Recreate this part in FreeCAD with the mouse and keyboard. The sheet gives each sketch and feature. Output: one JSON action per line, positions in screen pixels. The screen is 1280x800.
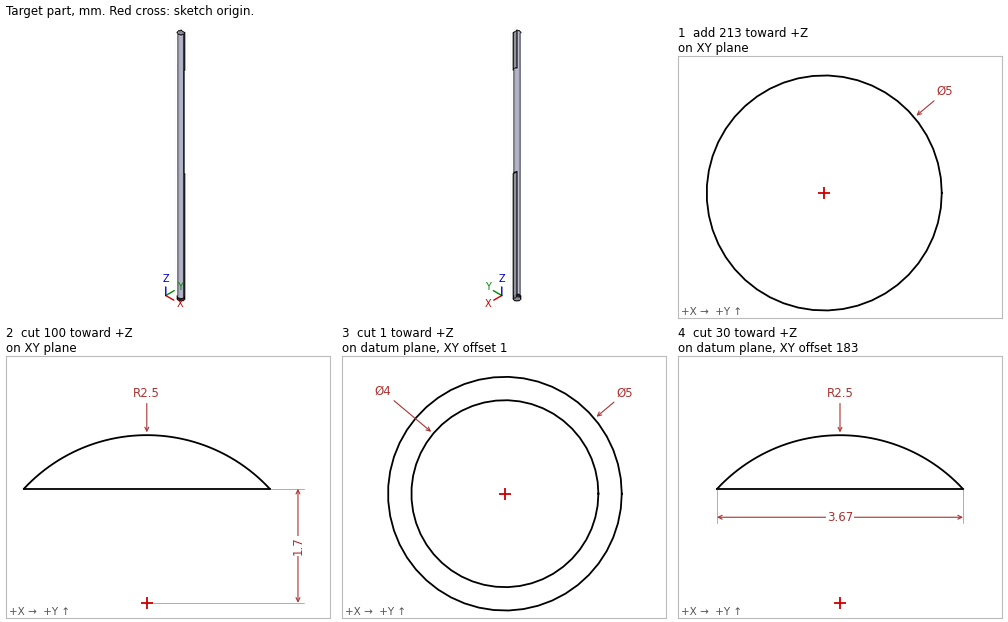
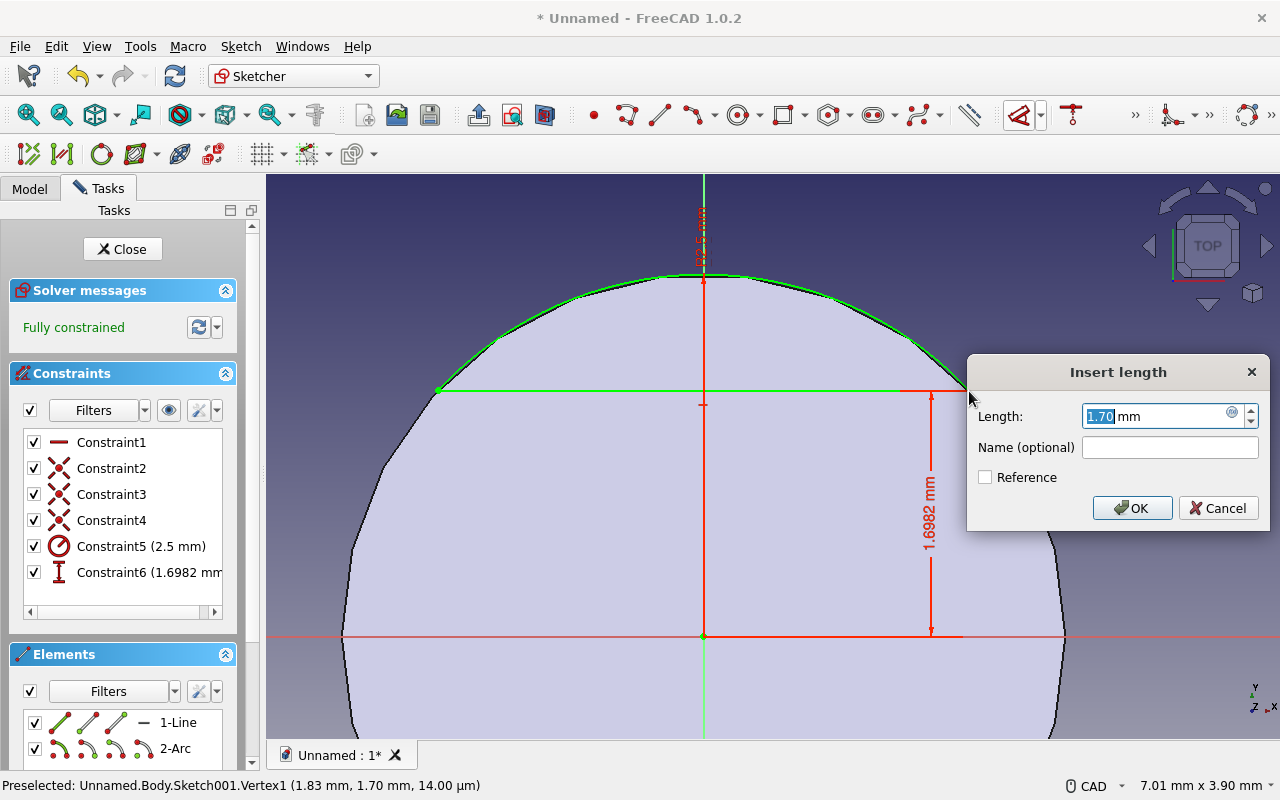
{"action": "type", "text": "1.7"}
{"action": "key", "text": "Return"}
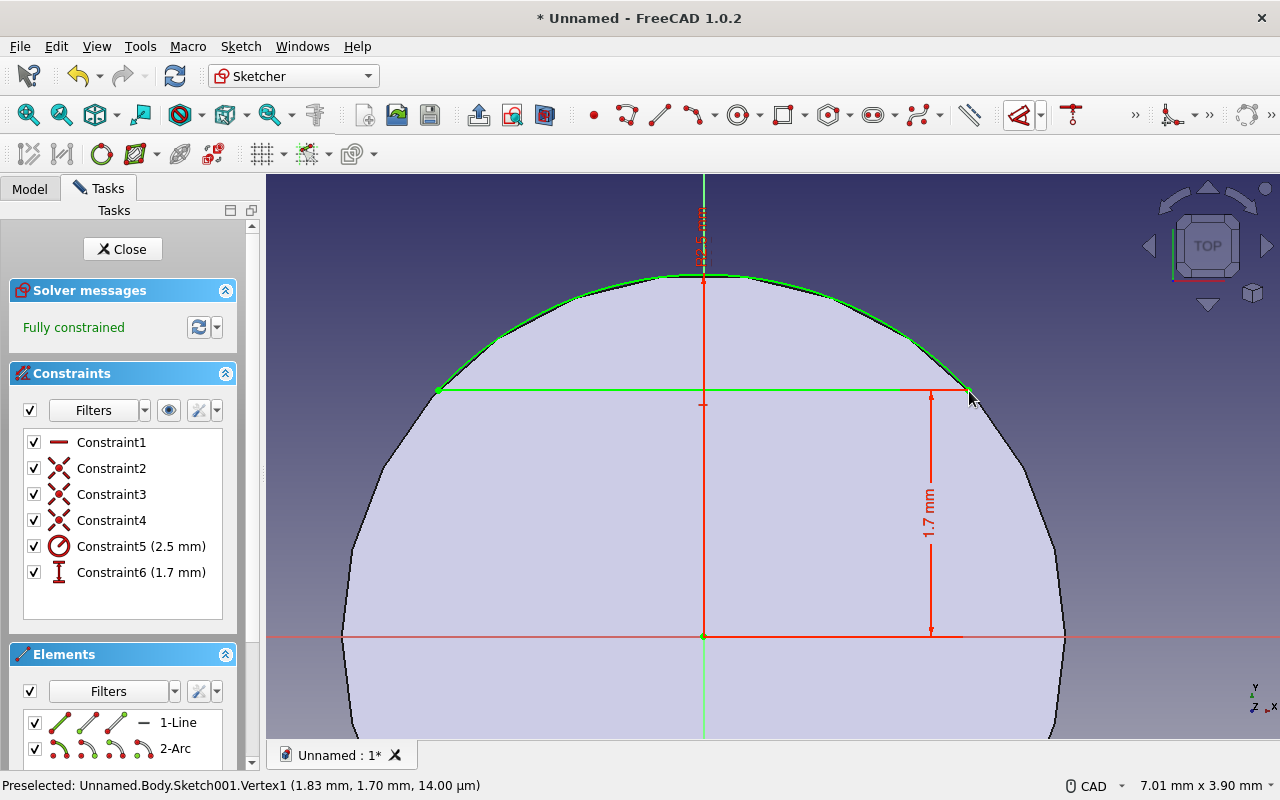
{"action": "left_click", "coordinate": [123, 249]}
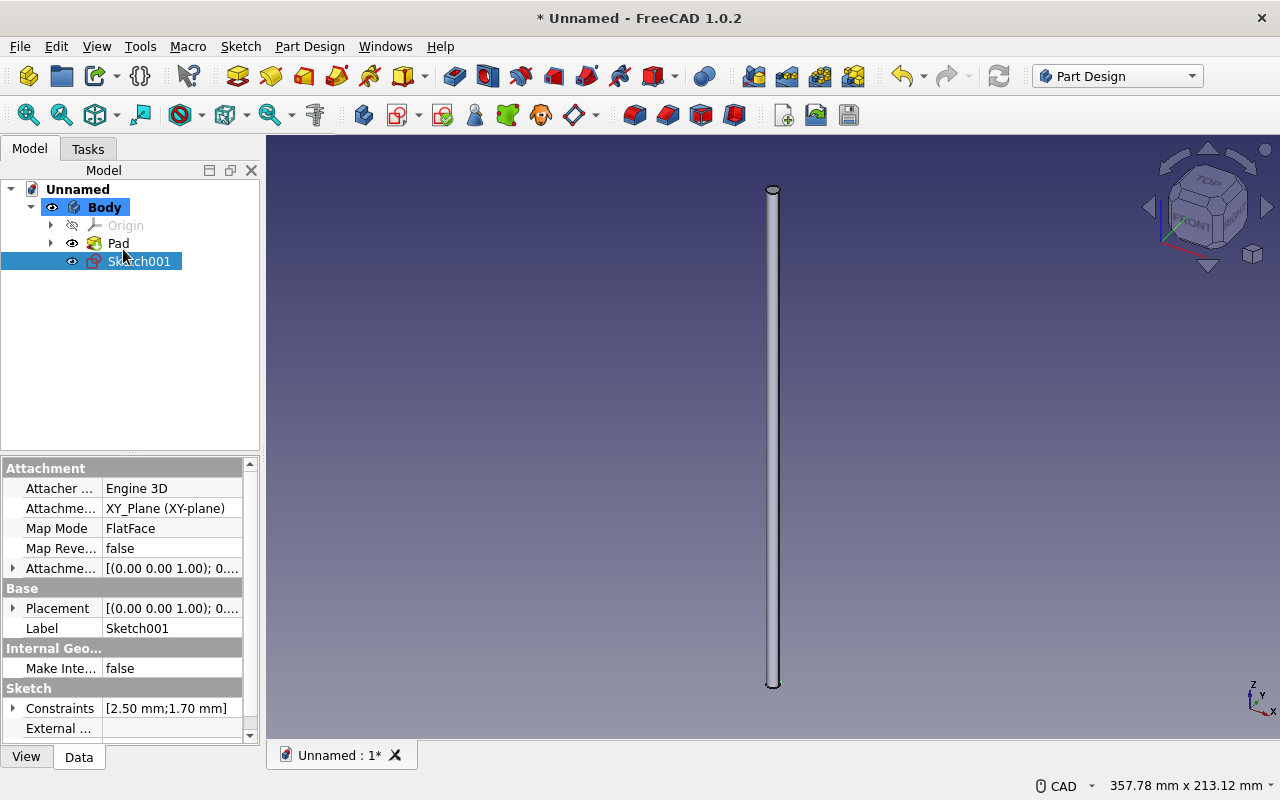
{"action": "left_click", "coordinate": [455, 76]}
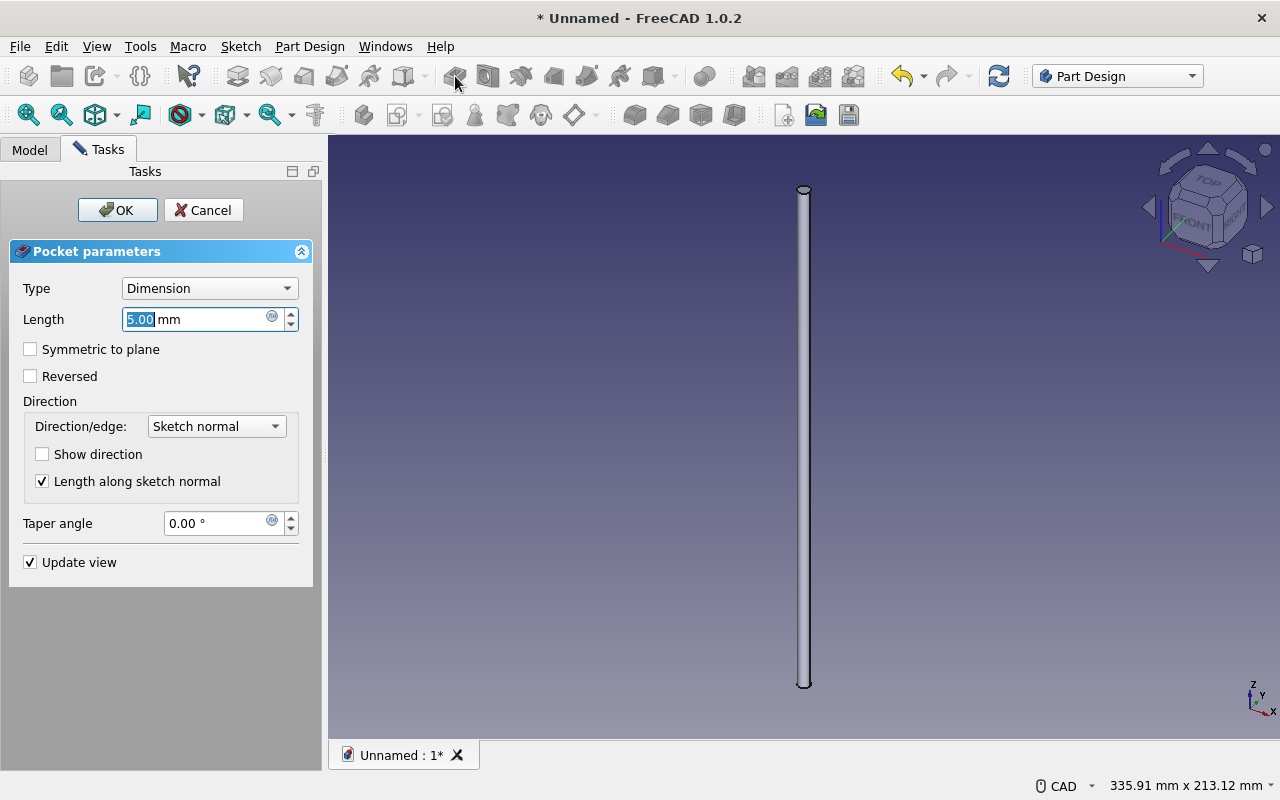
{"action": "type", "text": "100"}
{"action": "key", "text": "Tab"}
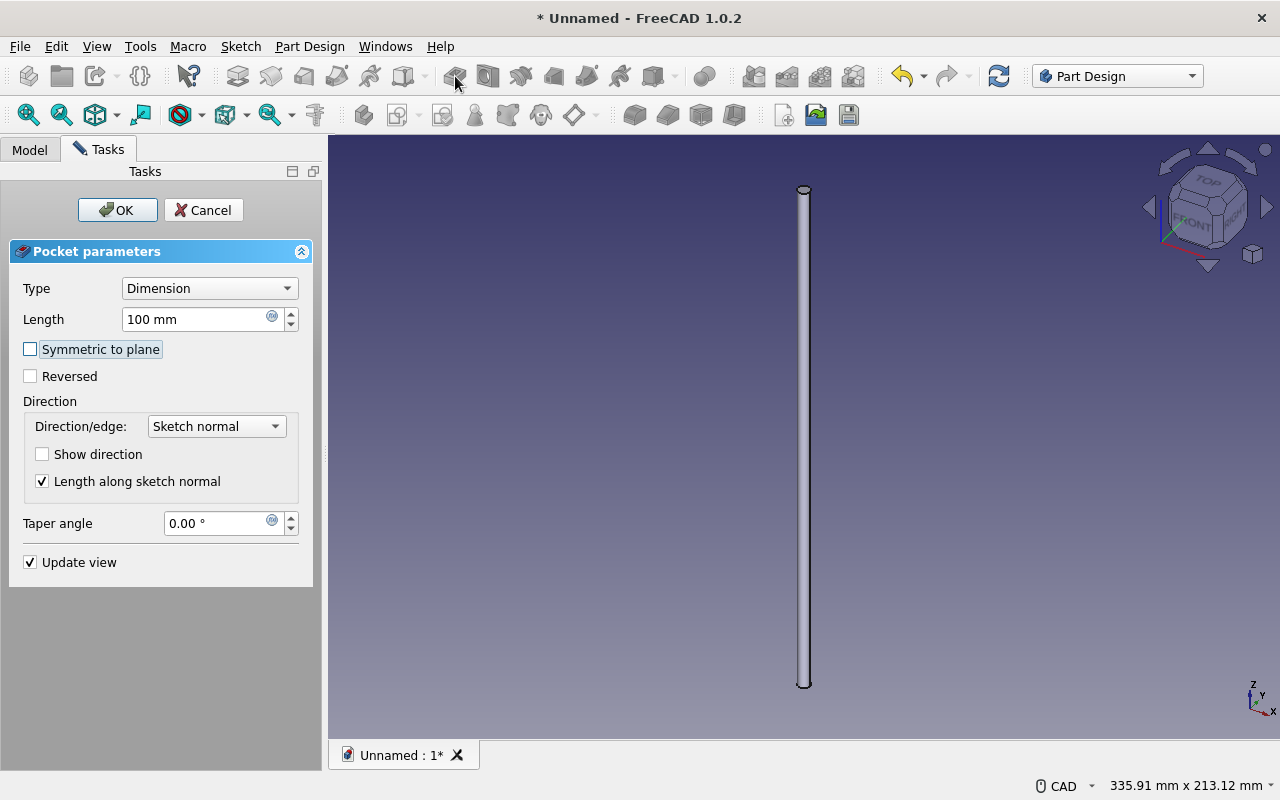
{"action": "left_click", "coordinate": [31, 376]}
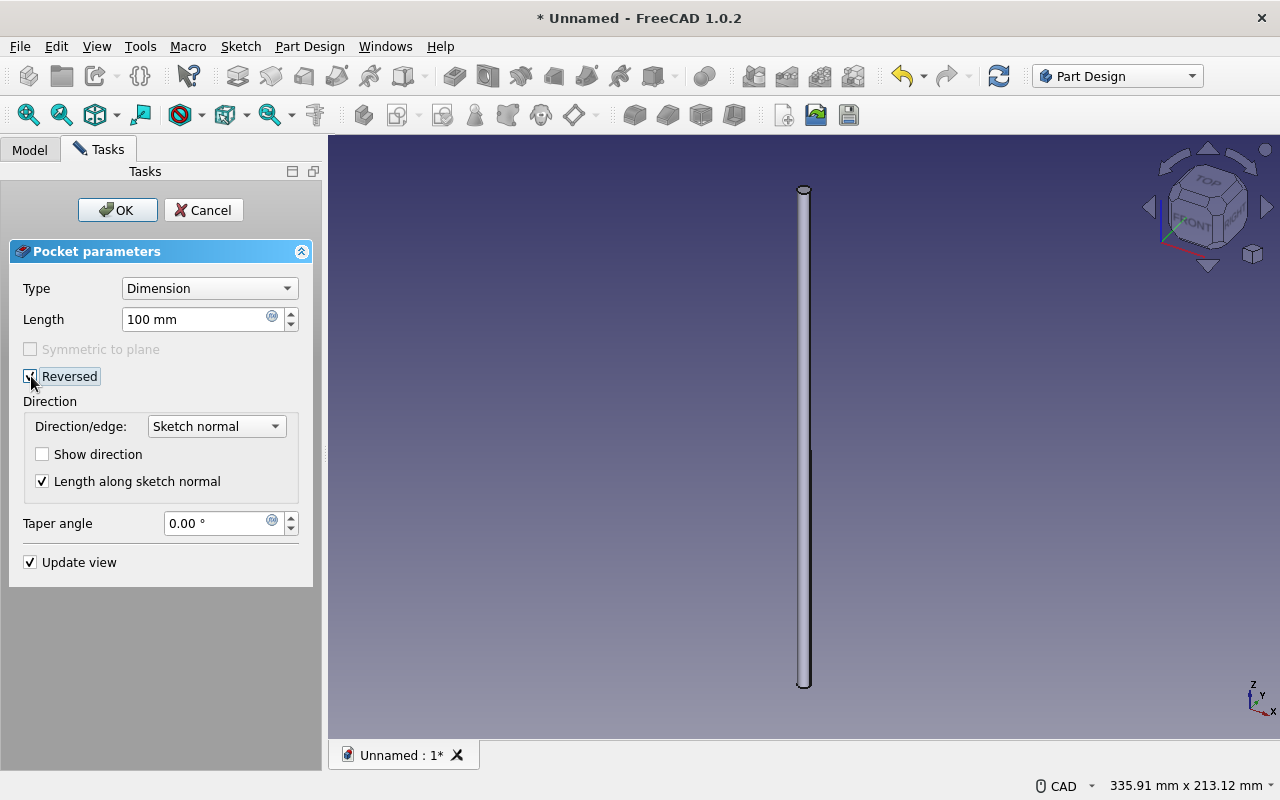
{"action": "left_click", "coordinate": [118, 210]}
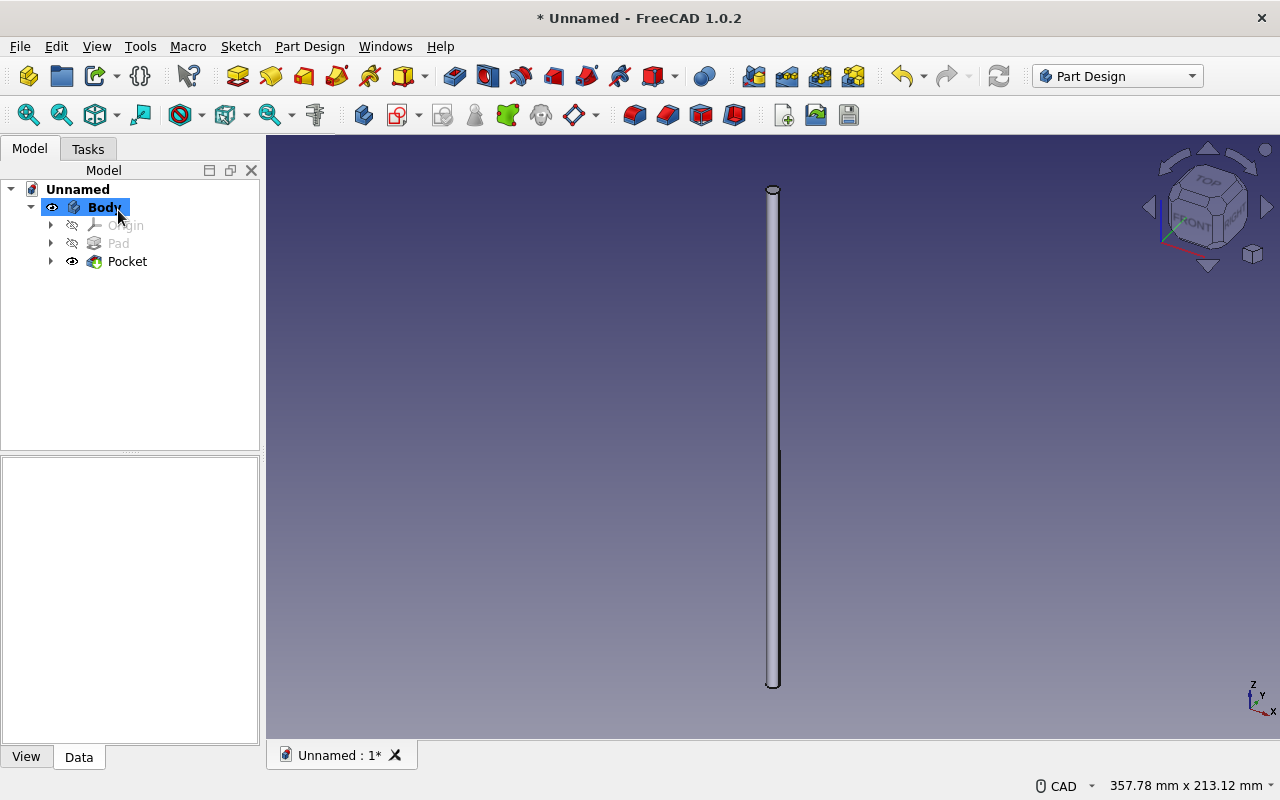
{"action": "left_click", "coordinate": [51, 225]}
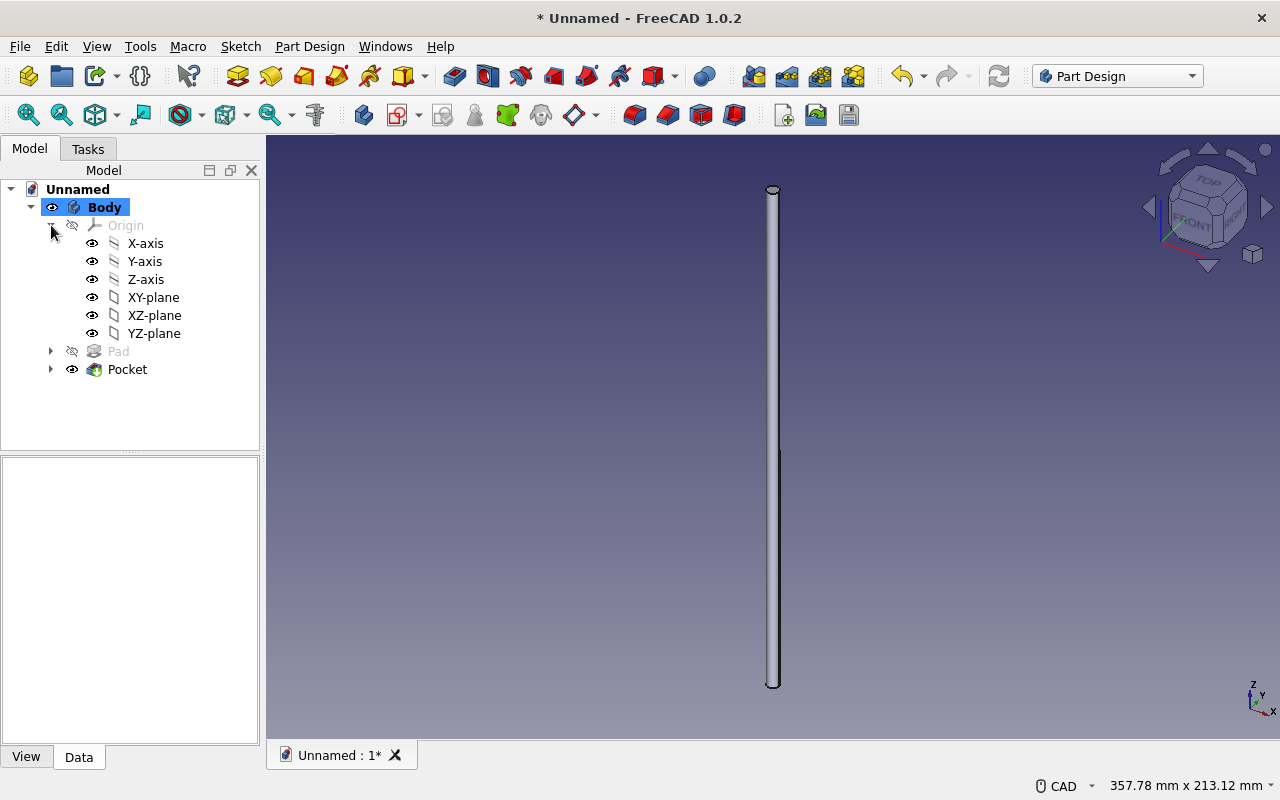
{"action": "left_click", "coordinate": [137, 297]}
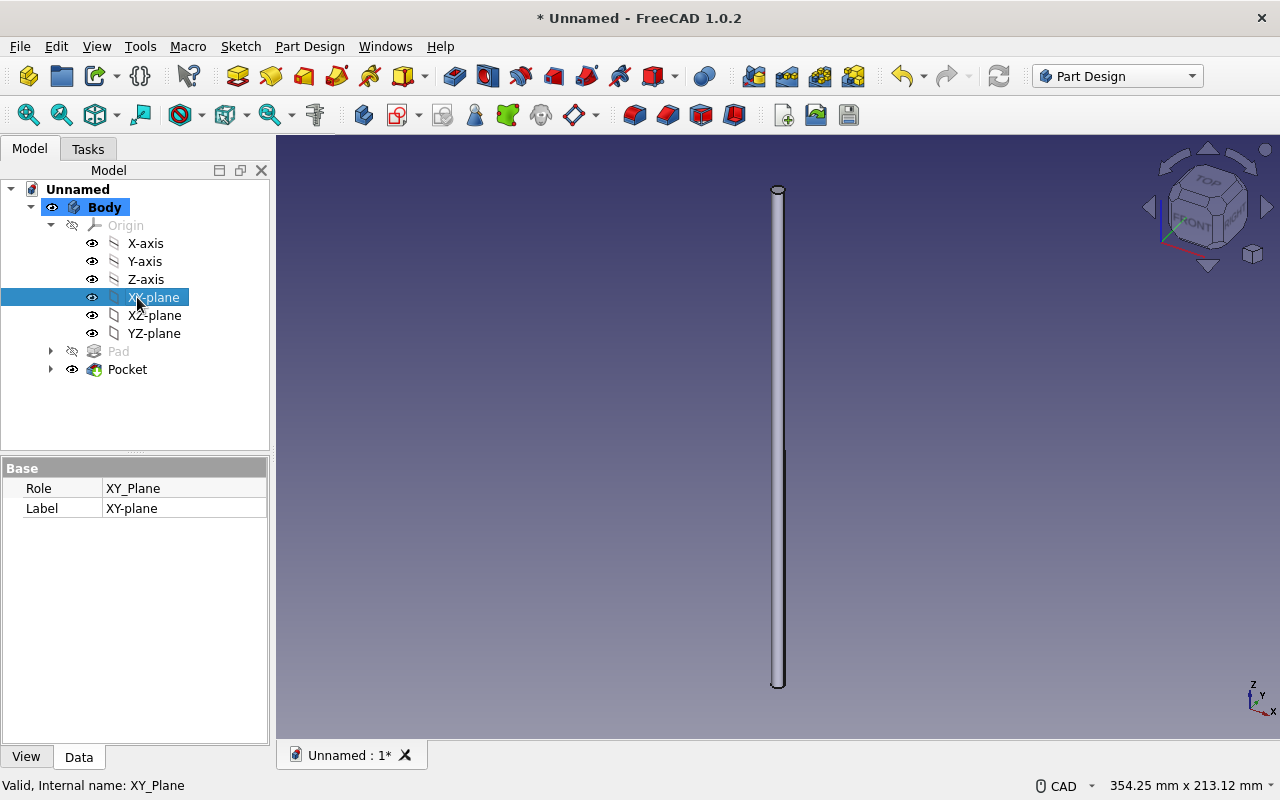
{"action": "left_click", "coordinate": [574, 116]}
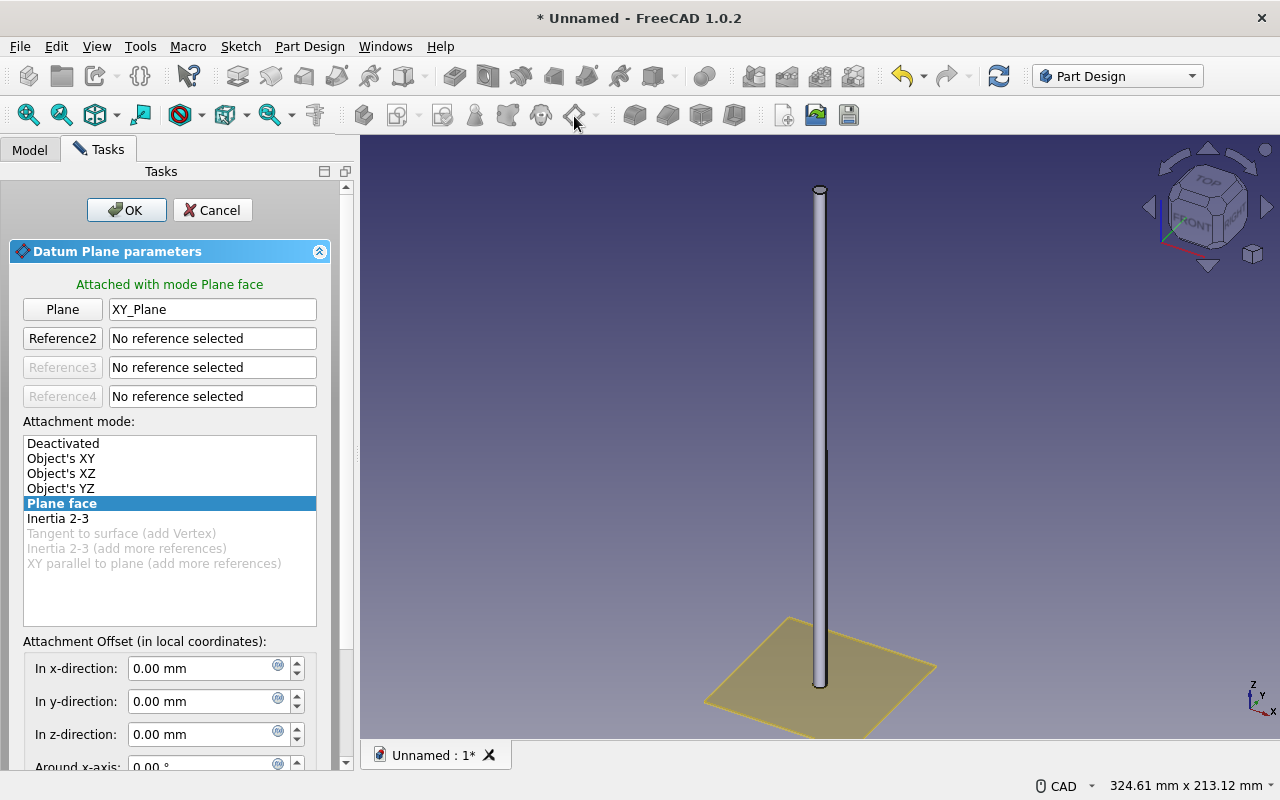
{"action": "triple_click", "coordinate": [210, 734]}